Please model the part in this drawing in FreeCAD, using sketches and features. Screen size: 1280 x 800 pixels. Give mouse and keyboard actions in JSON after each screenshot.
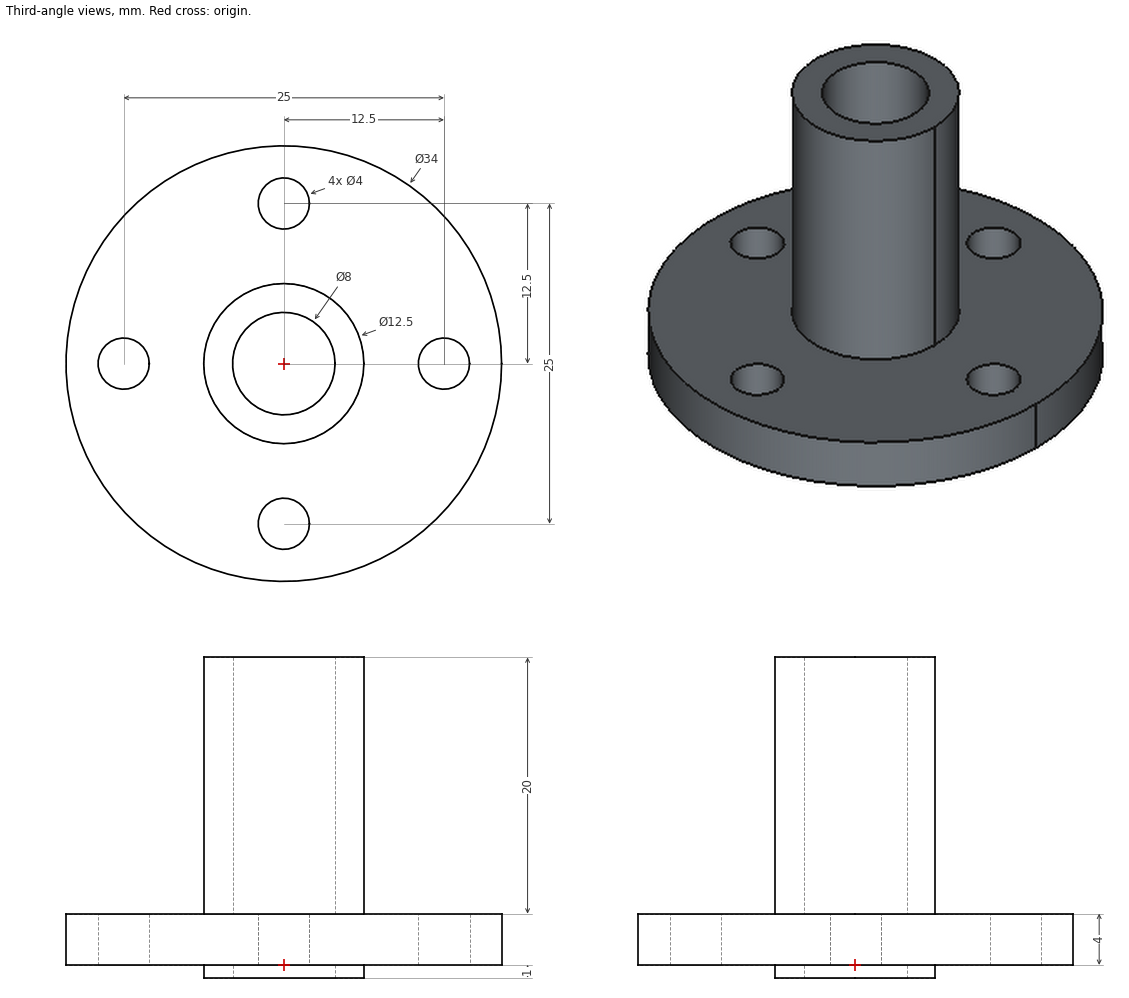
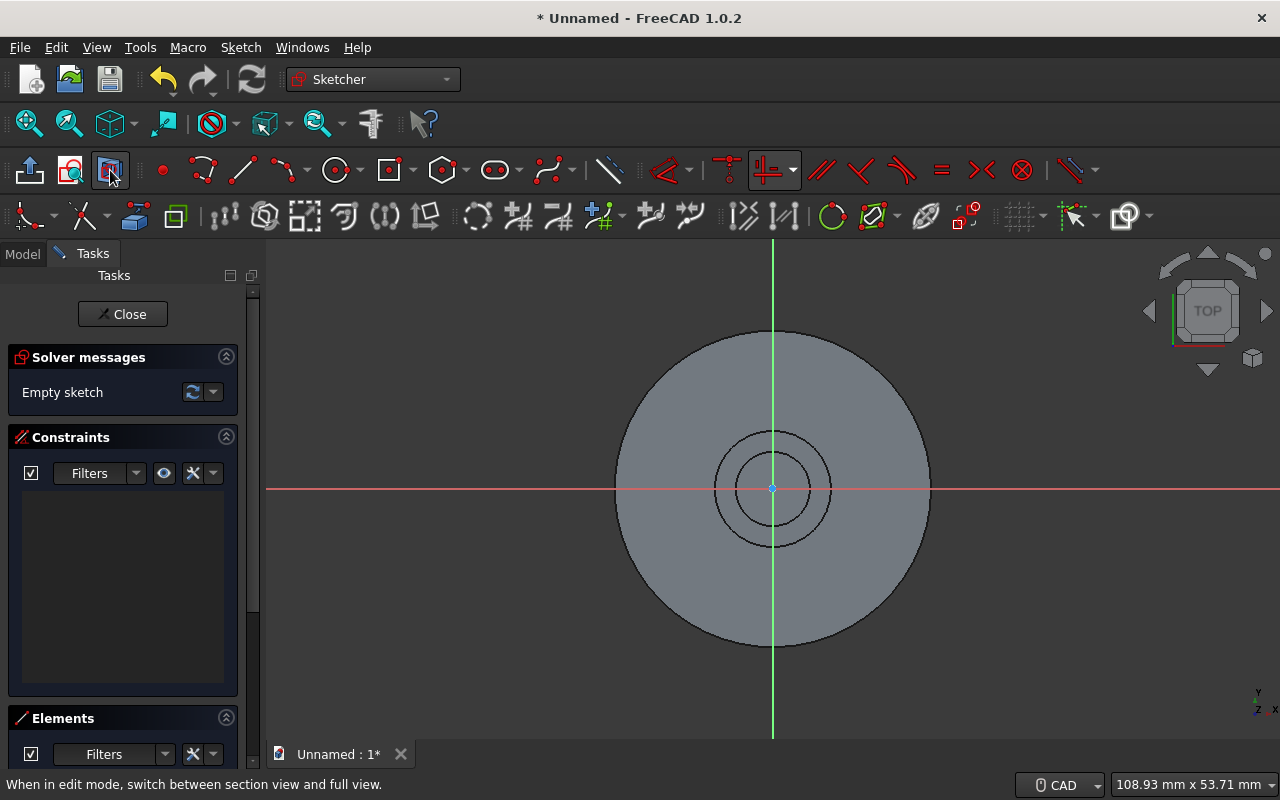
{"action": "left_click", "coordinate": [336, 170]}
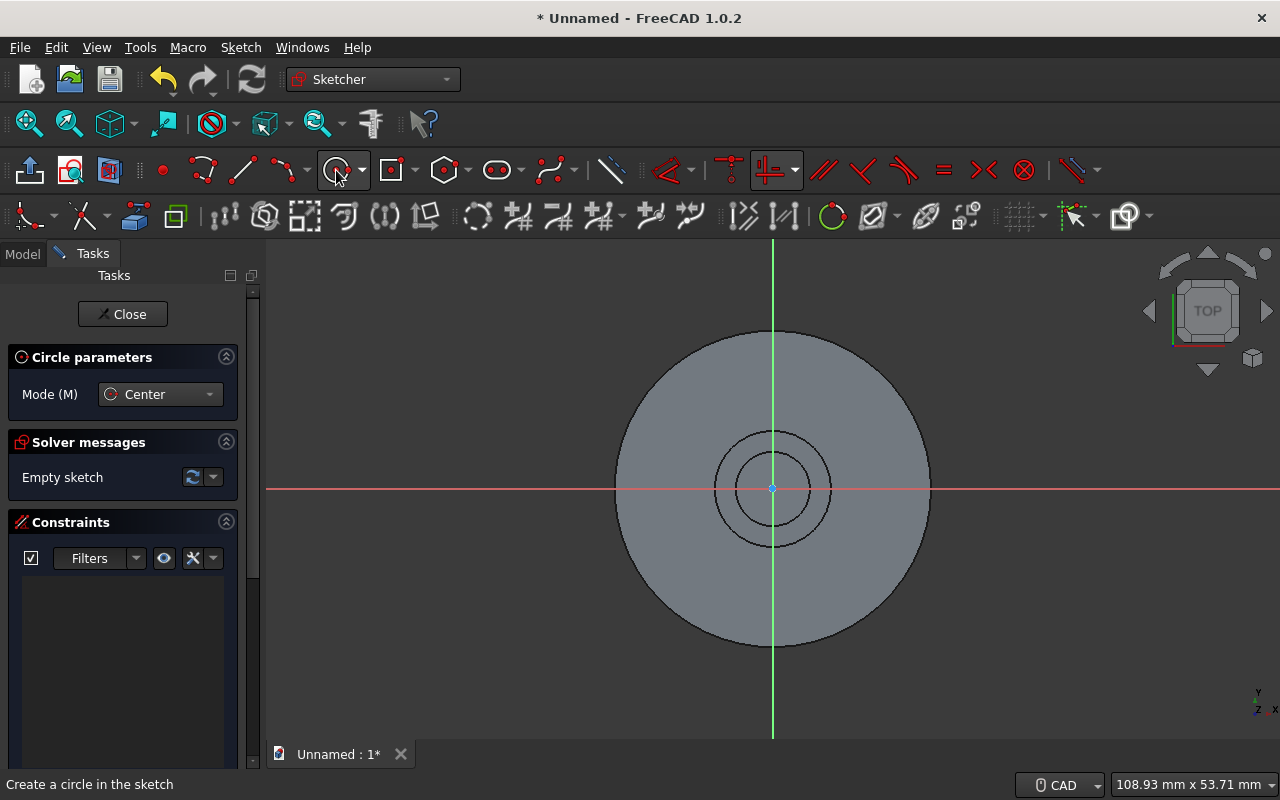
{"action": "left_click", "coordinate": [773, 373]}
{"action": "mouse_move", "coordinate": [790, 366]}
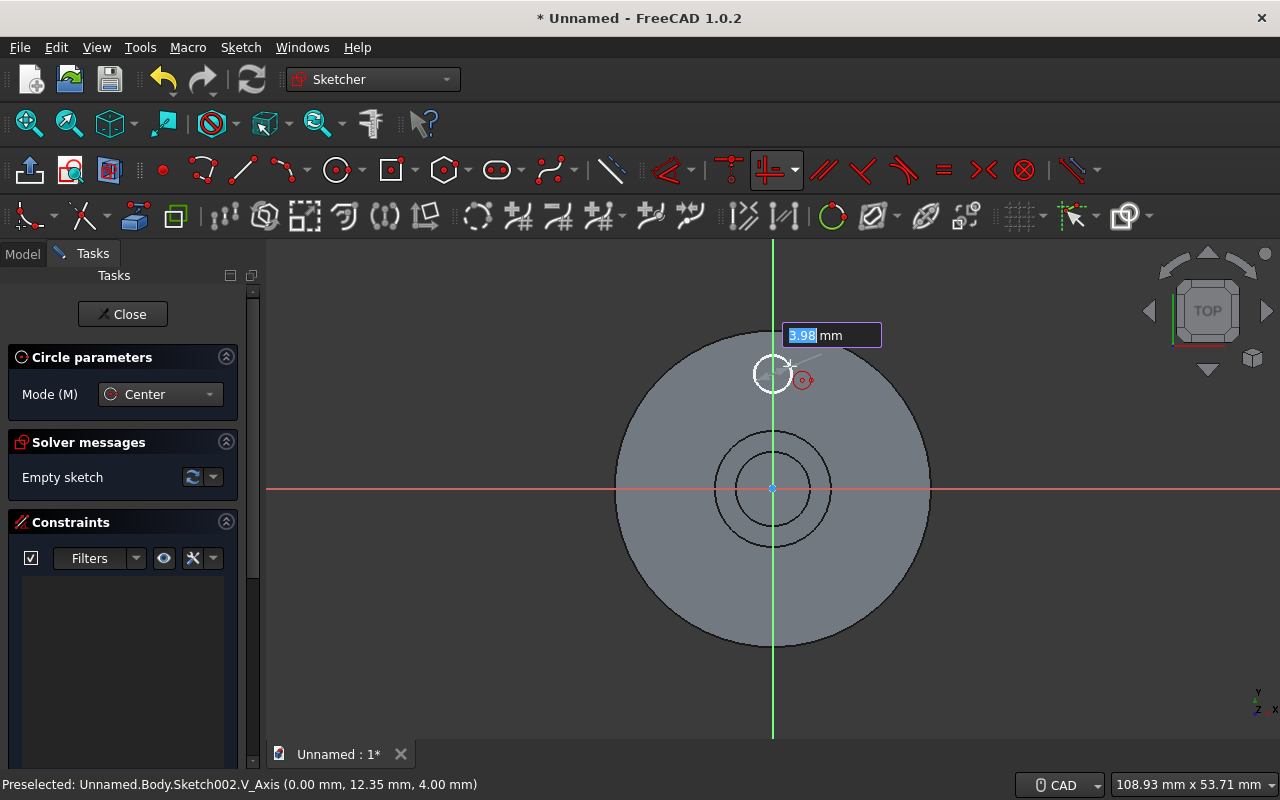
{"action": "type", "text": "4"}
{"action": "key", "text": "Return"}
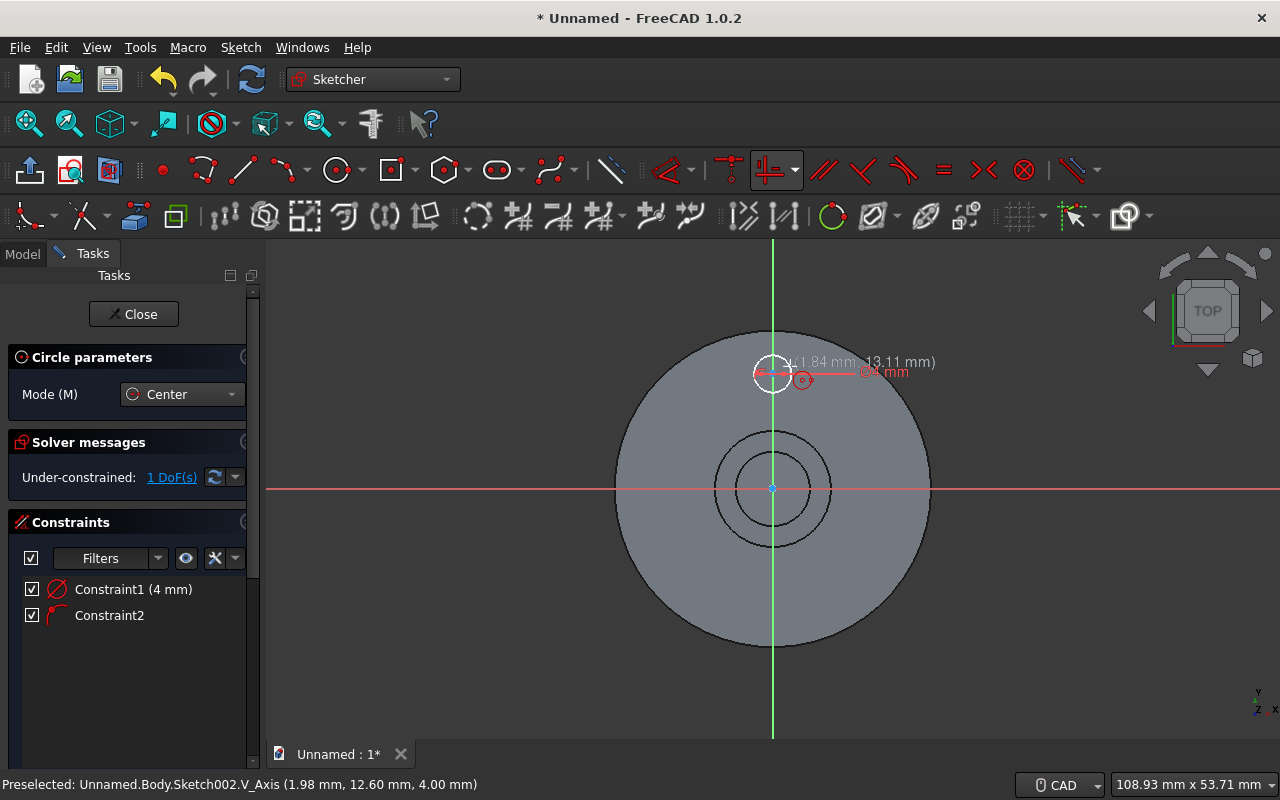
{"action": "left_click", "coordinate": [889, 489]}
{"action": "mouse_move", "coordinate": [896, 472]}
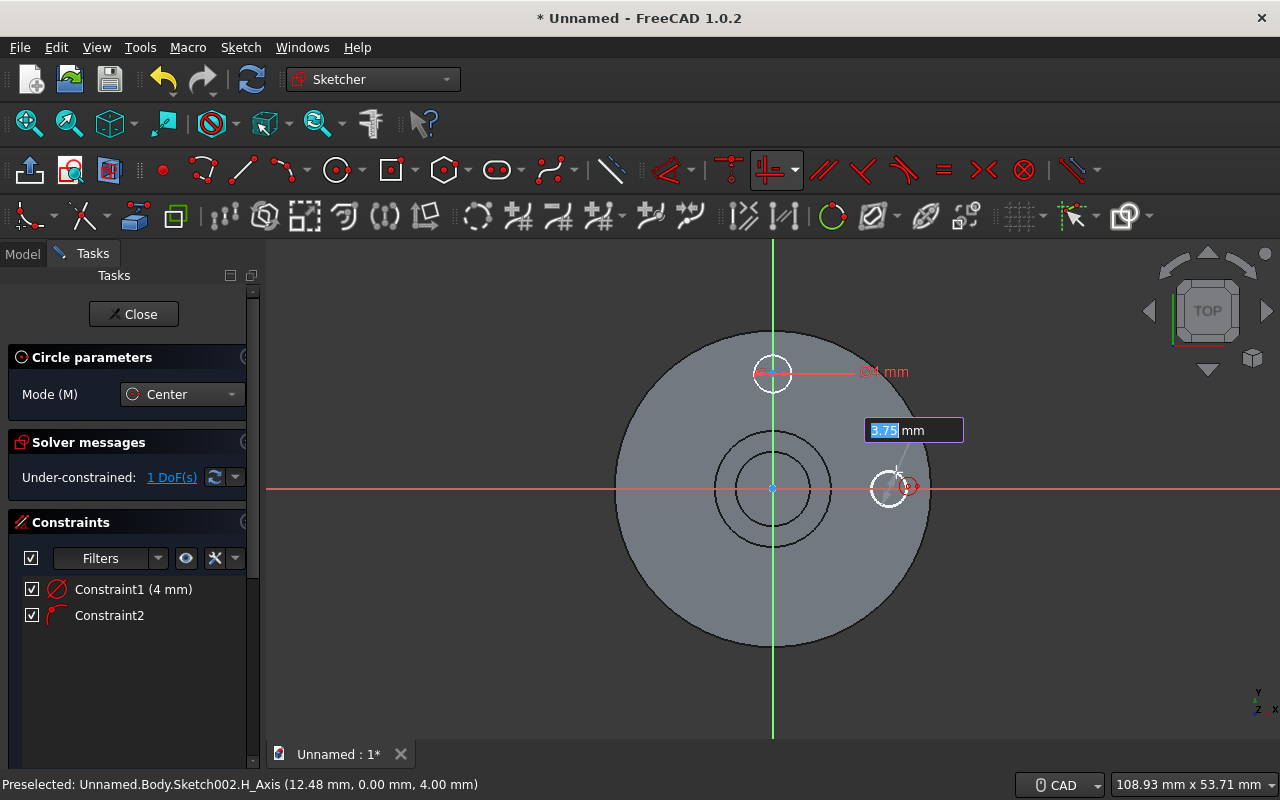
{"action": "type", "text": "4"}
{"action": "key", "text": "Return"}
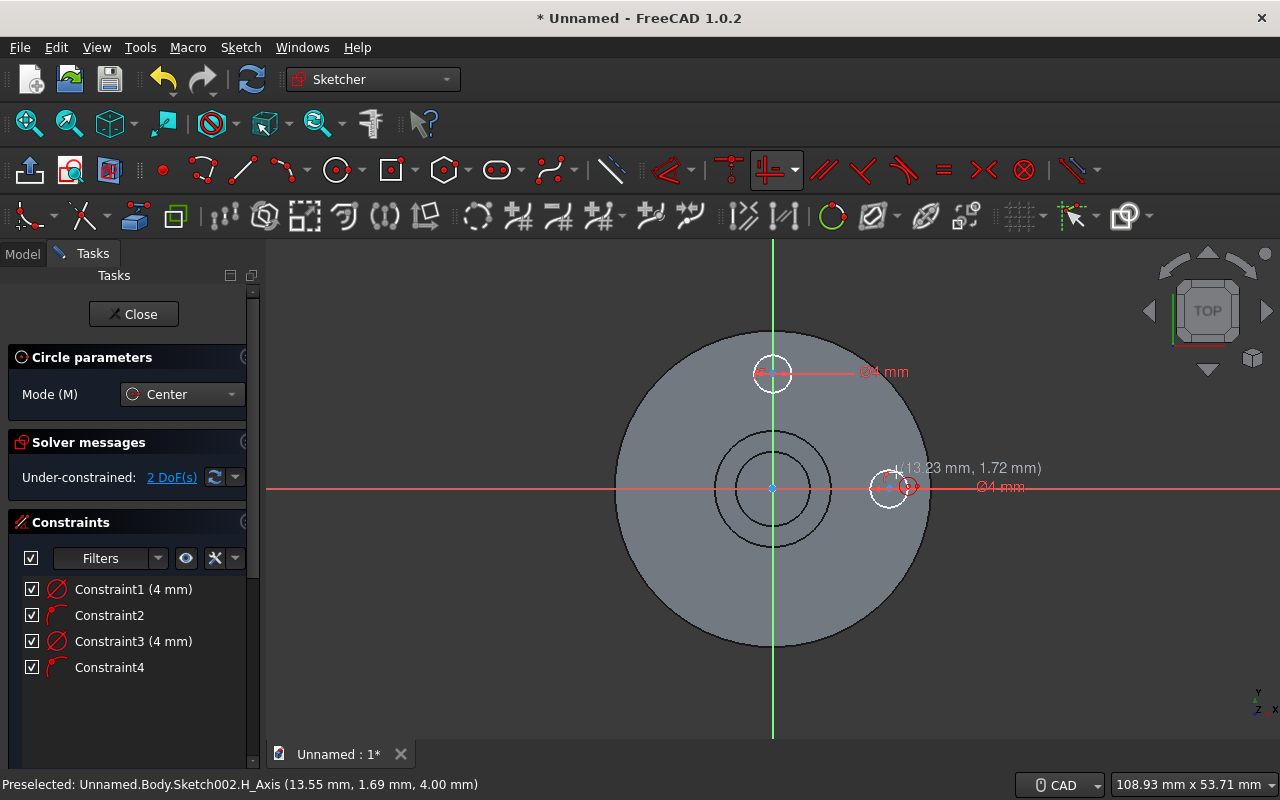
{"action": "left_click", "coordinate": [773, 605]}
{"action": "mouse_move", "coordinate": [790, 599]}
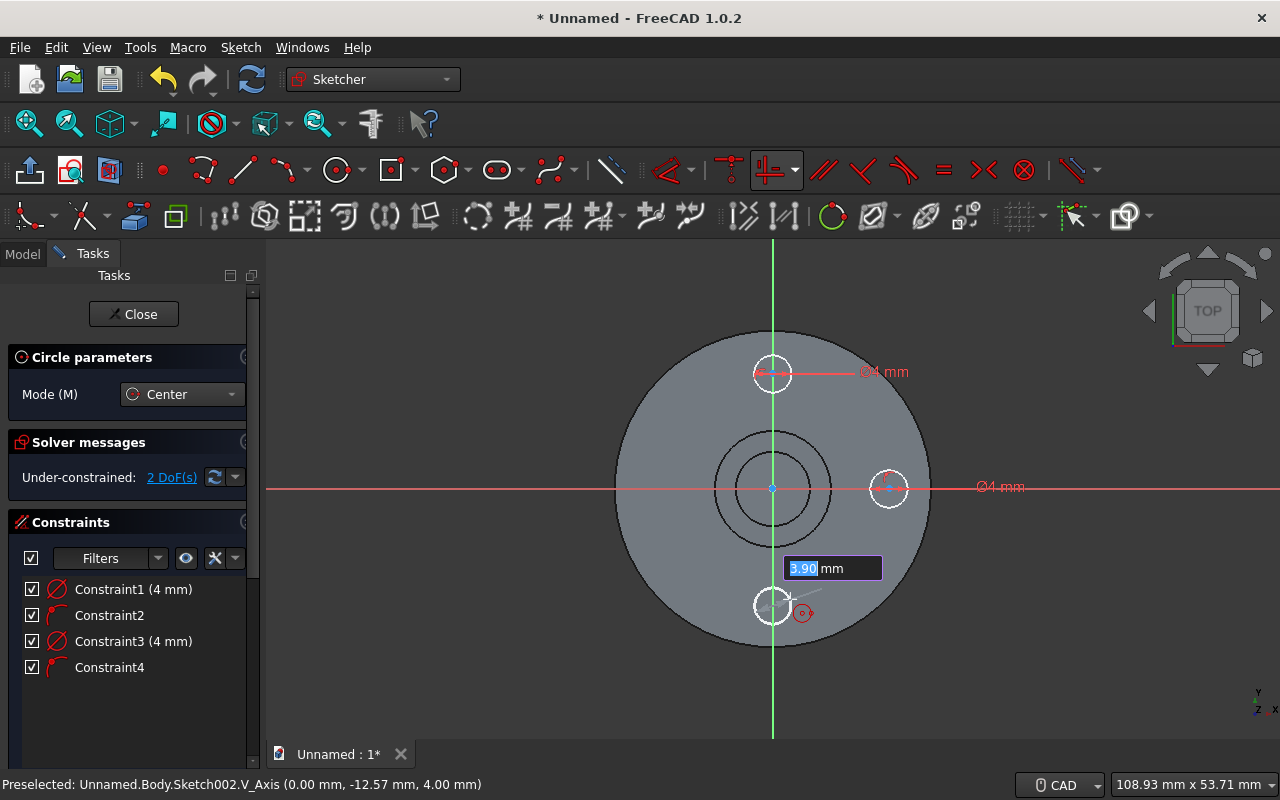
{"action": "type", "text": "4"}
{"action": "key", "text": "Return"}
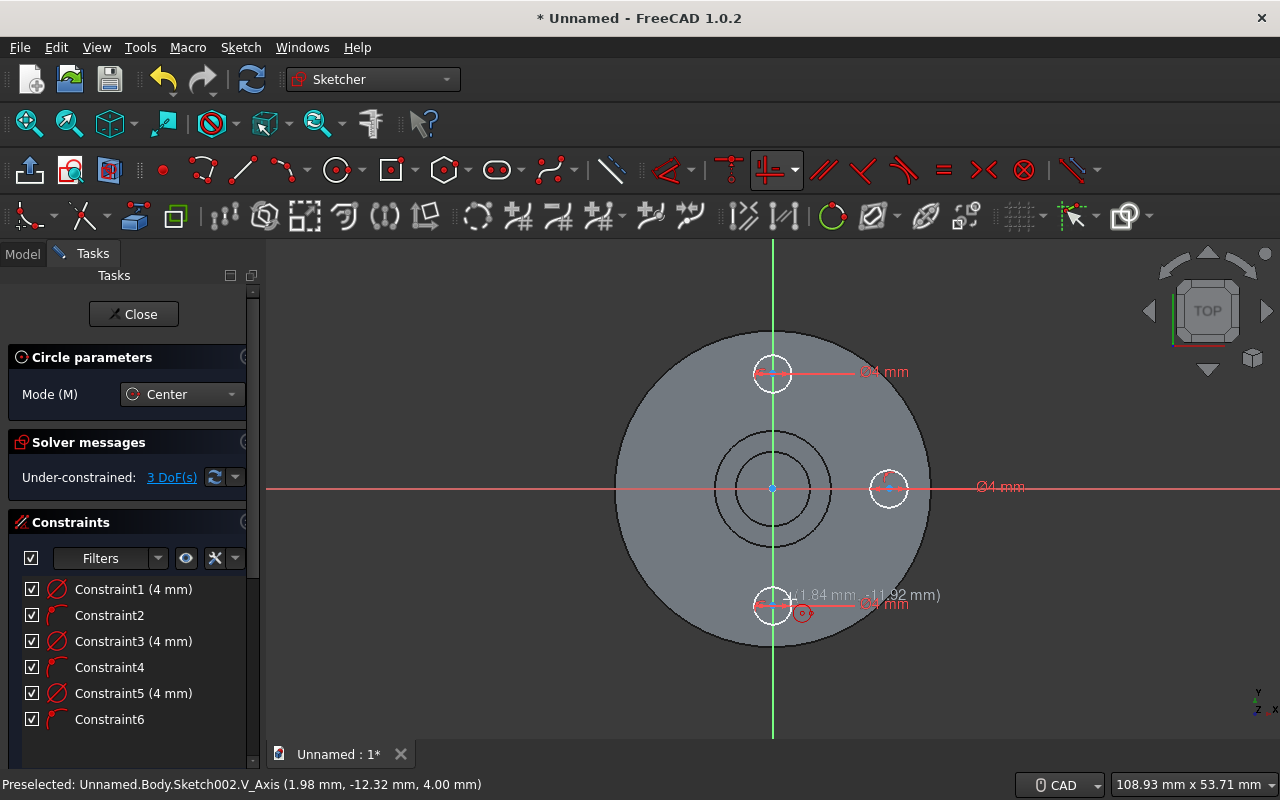
{"action": "left_click", "coordinate": [656, 489]}
{"action": "mouse_move", "coordinate": [663, 472]}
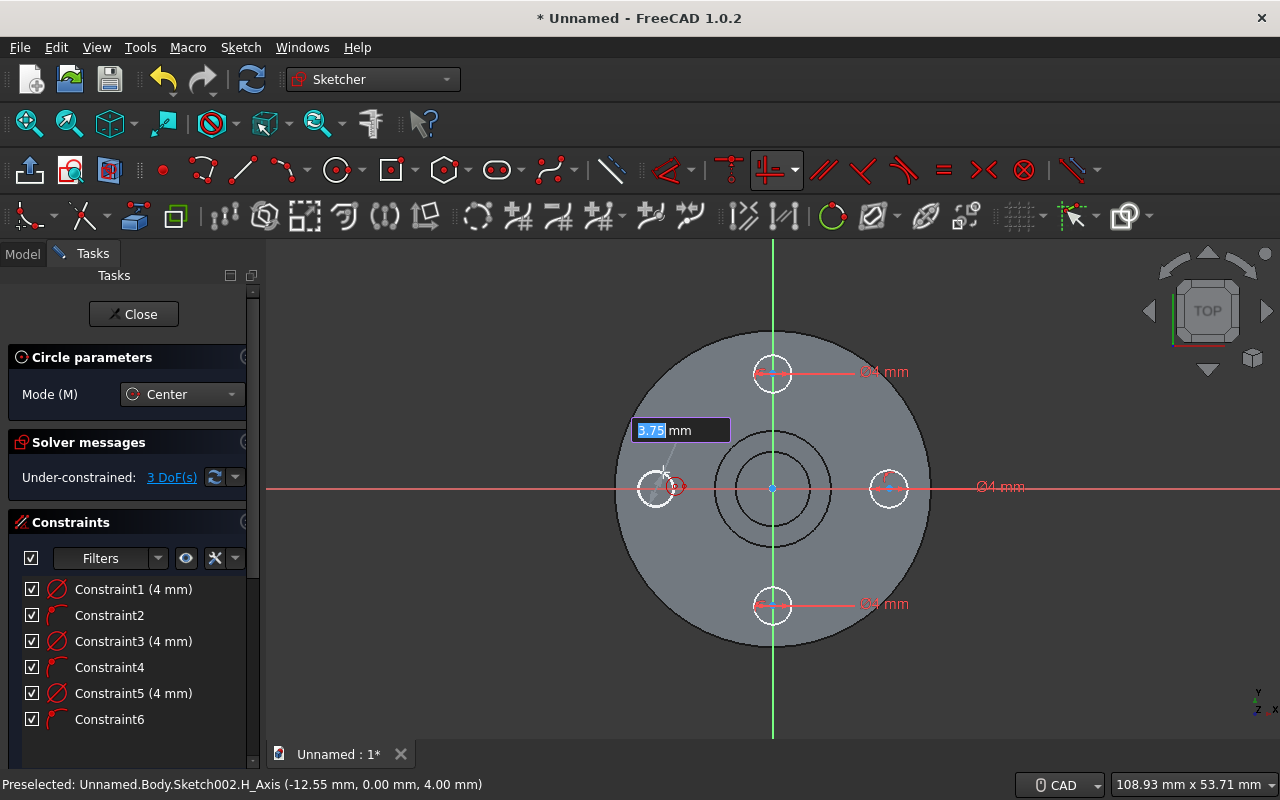
{"action": "type", "text": "4"}
{"action": "key", "text": "Return"}
{"action": "key", "text": "Escape"}